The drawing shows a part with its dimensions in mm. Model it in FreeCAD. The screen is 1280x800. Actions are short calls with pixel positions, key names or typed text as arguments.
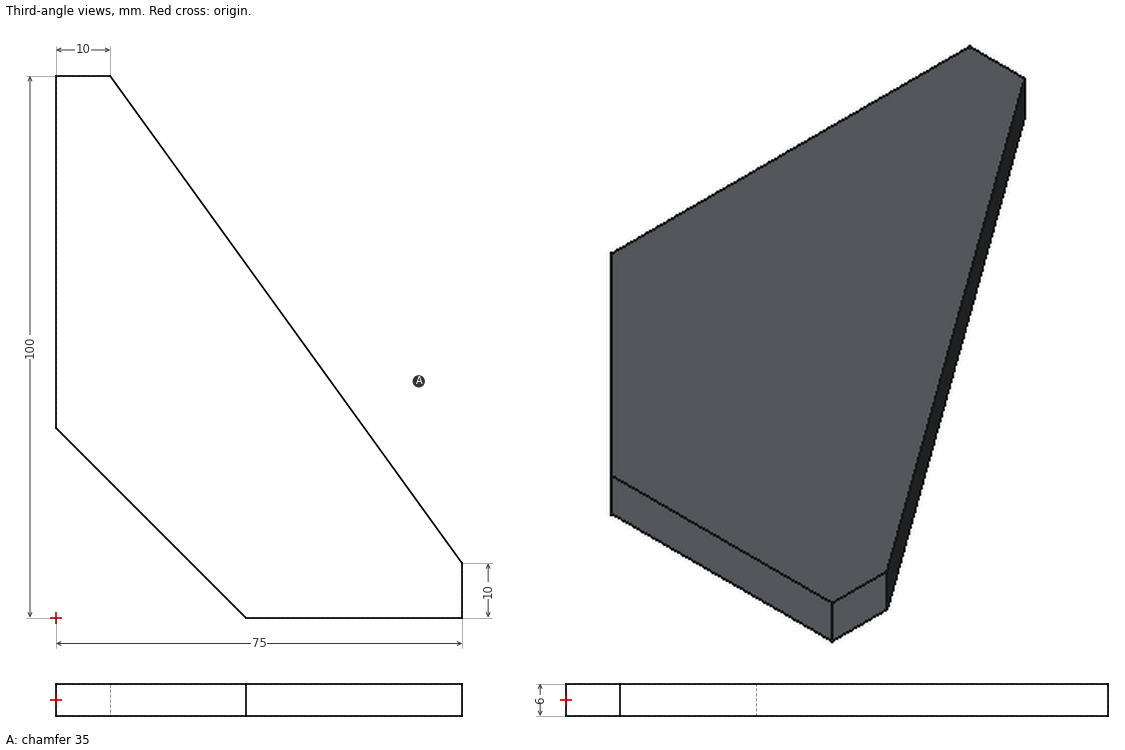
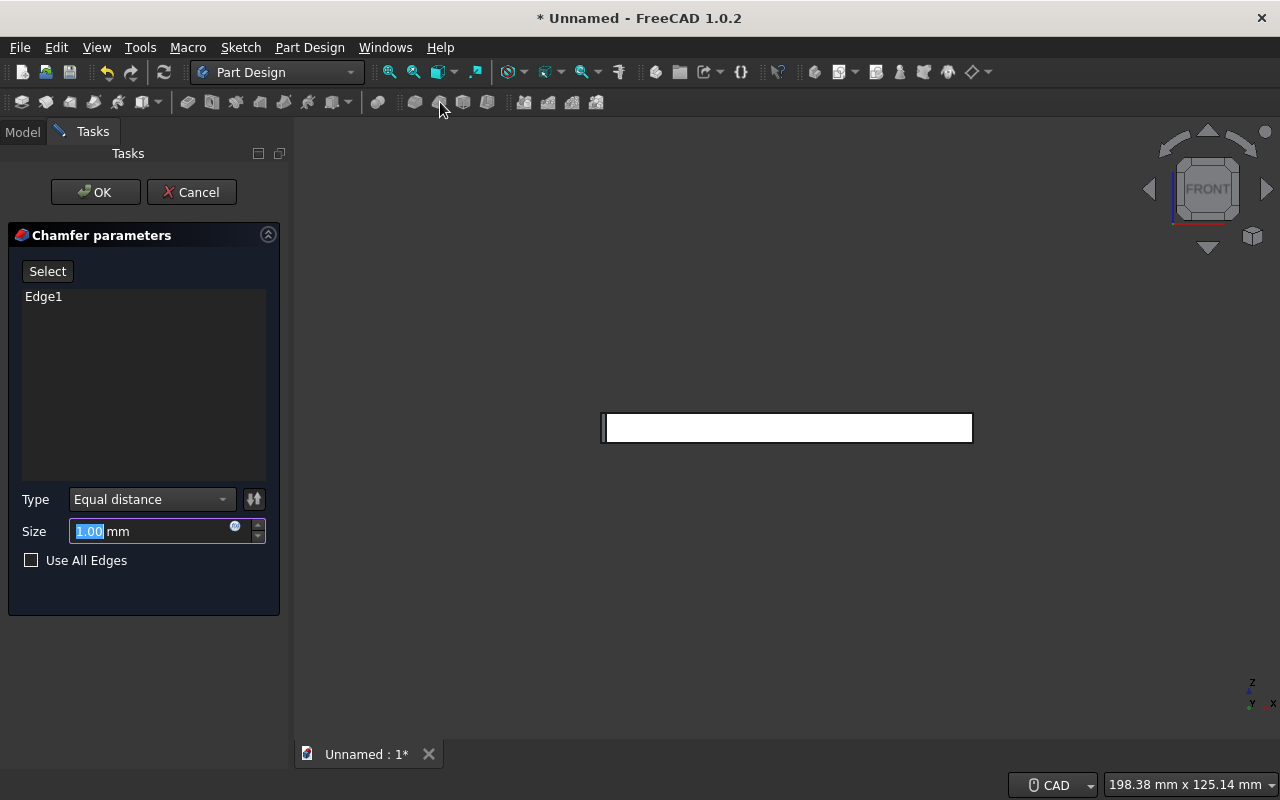
text(35)
key(Tab)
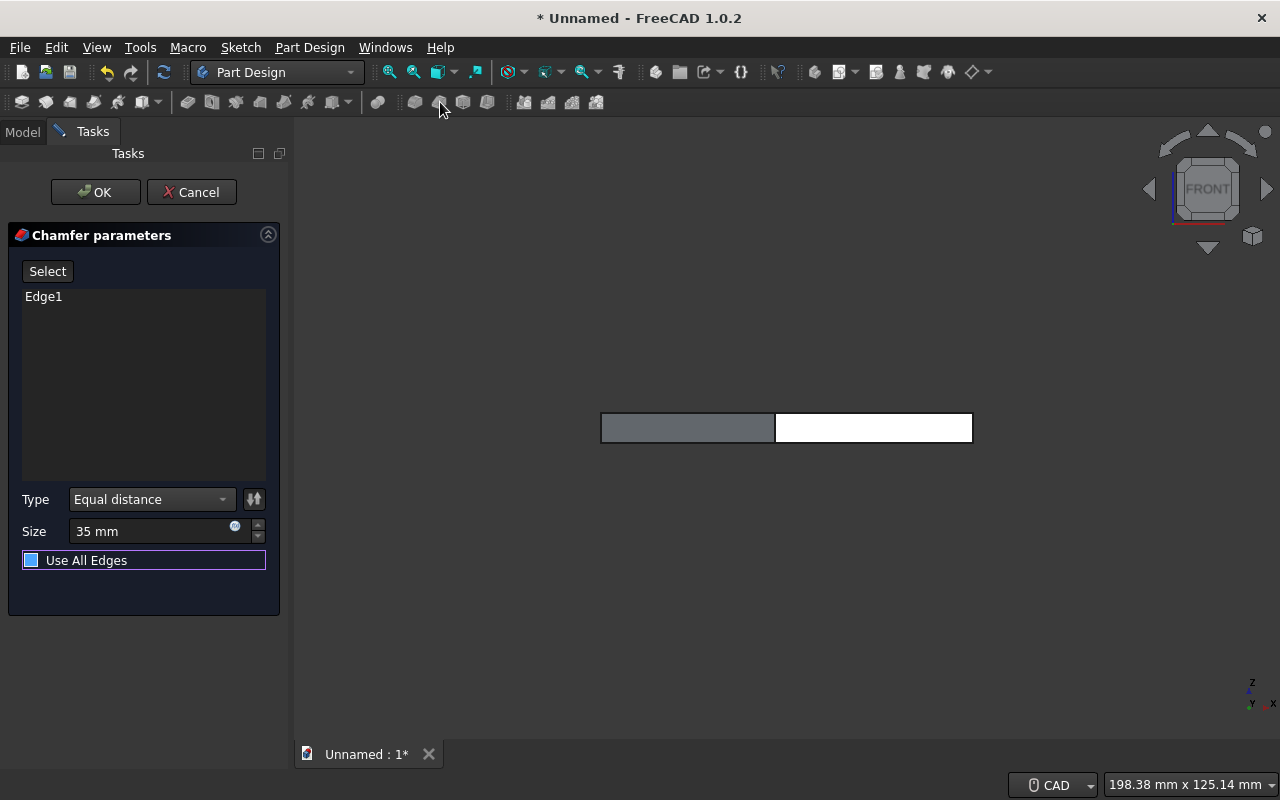
click(96, 192)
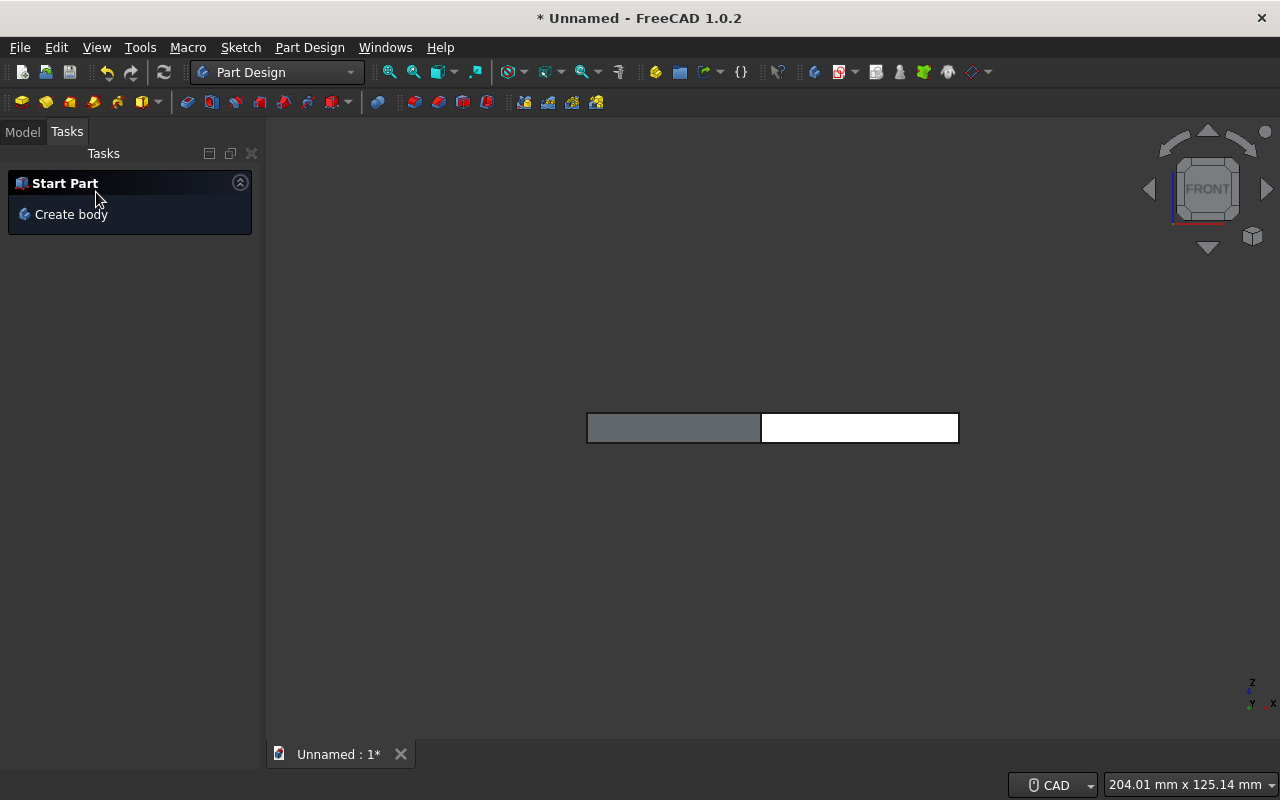
key(0)